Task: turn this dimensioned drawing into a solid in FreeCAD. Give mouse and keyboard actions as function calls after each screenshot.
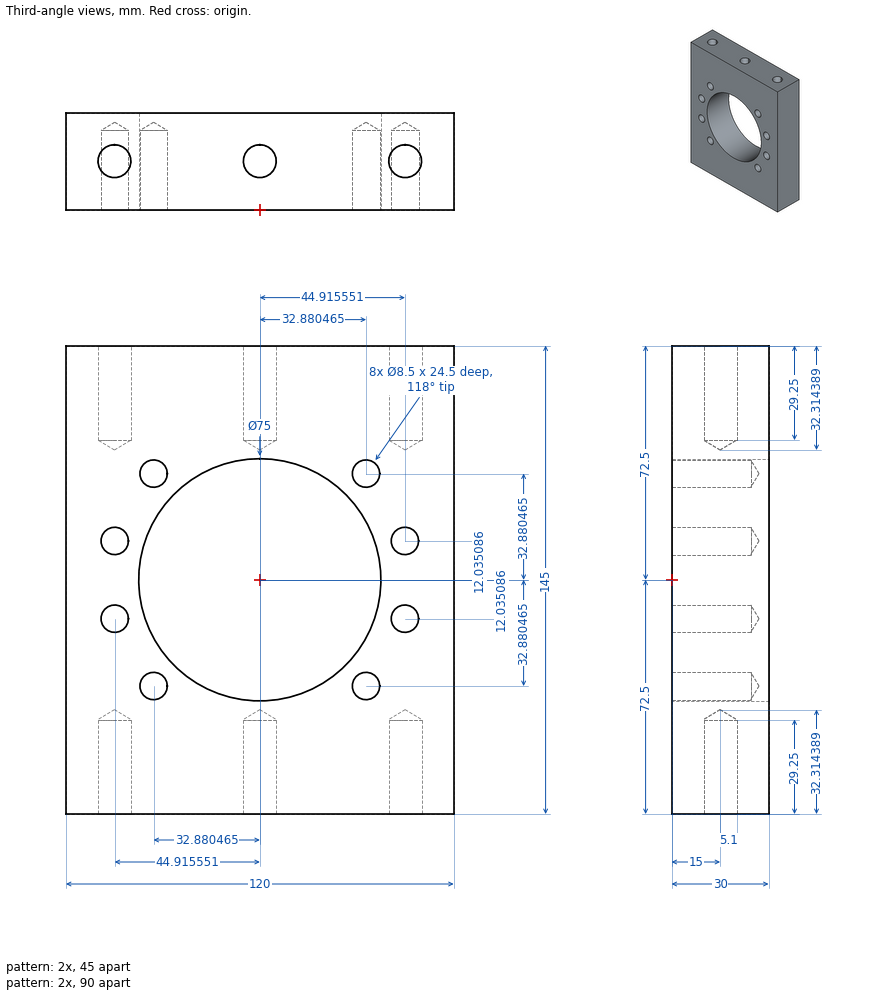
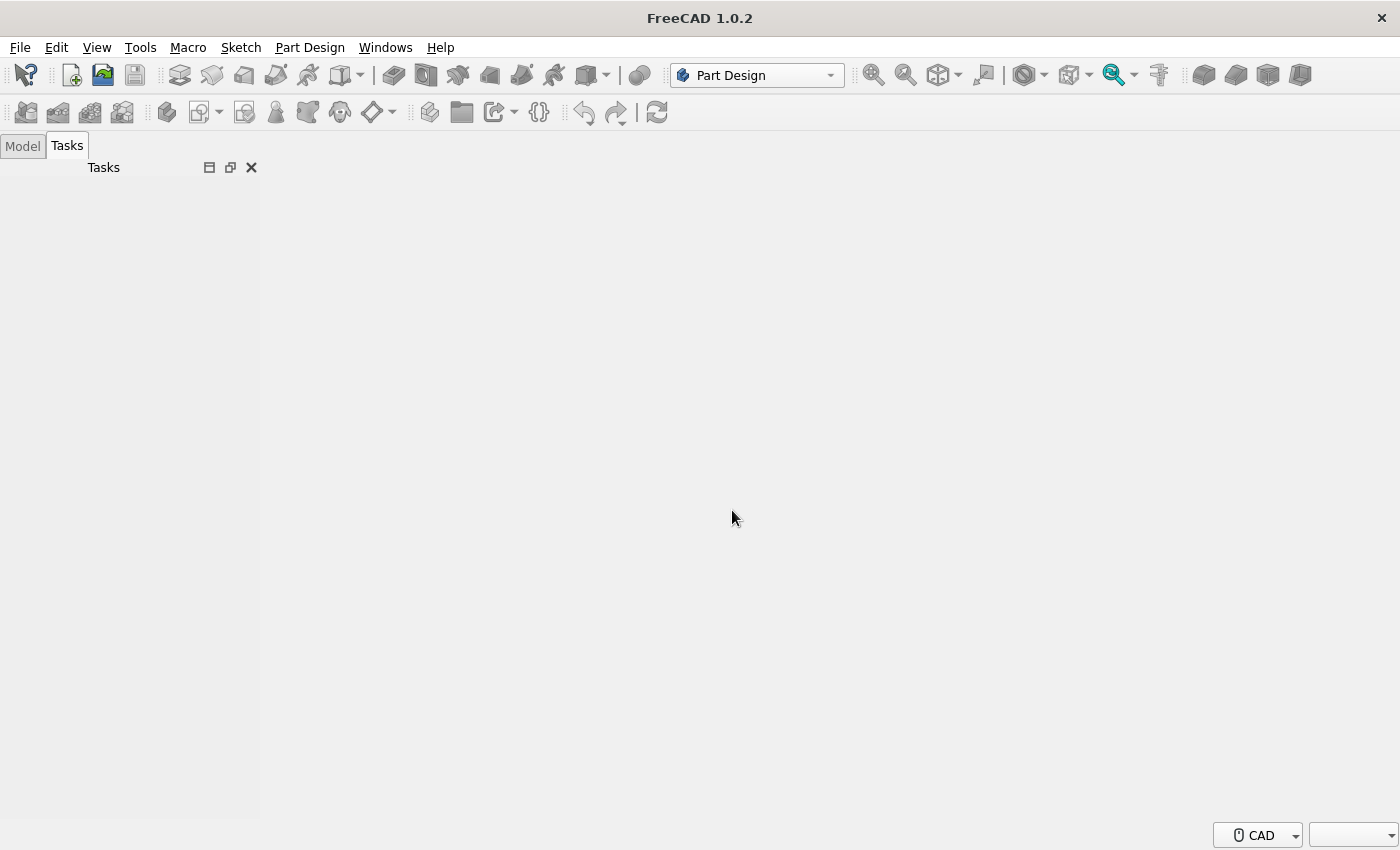
click(72, 76)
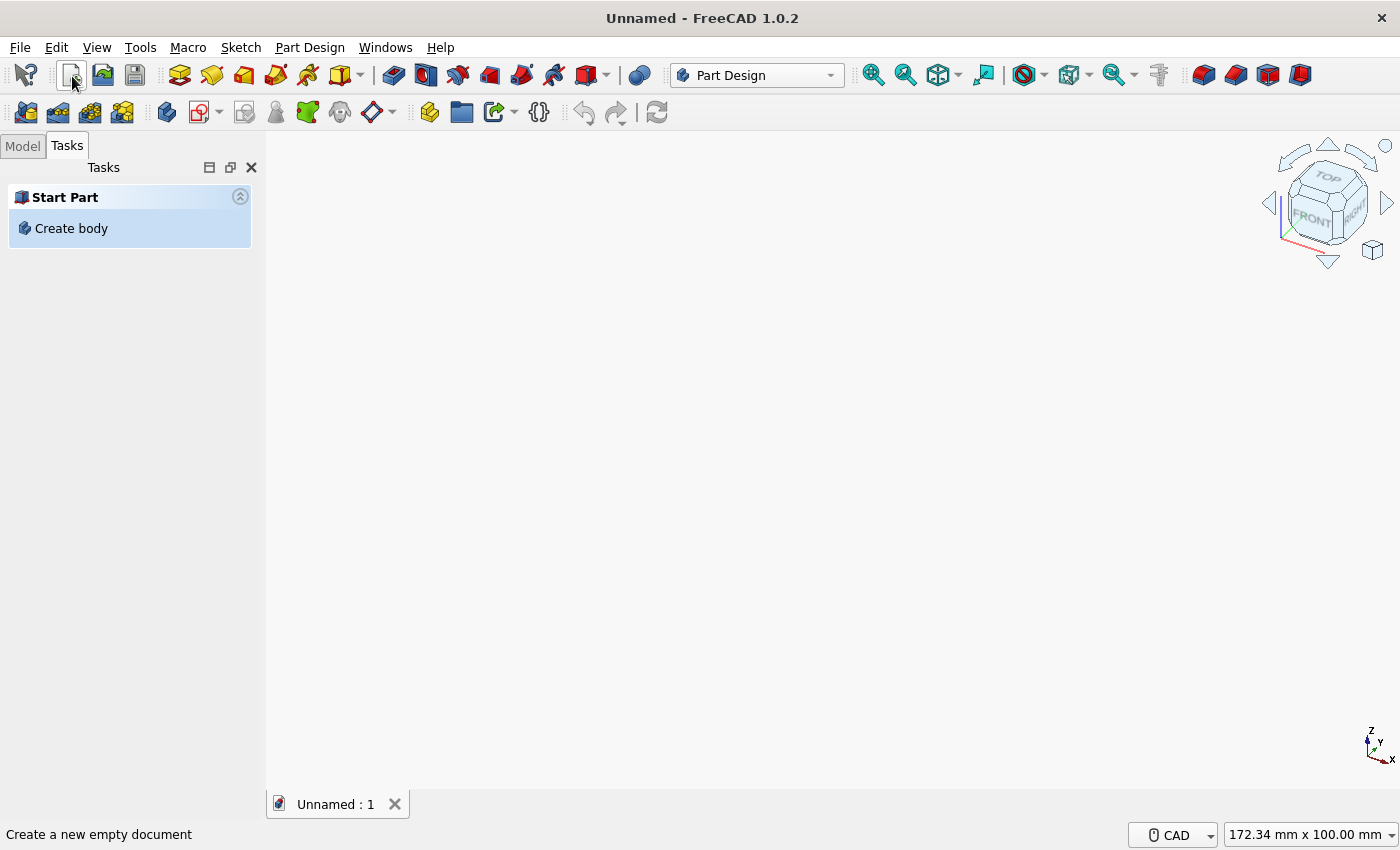
click(200, 112)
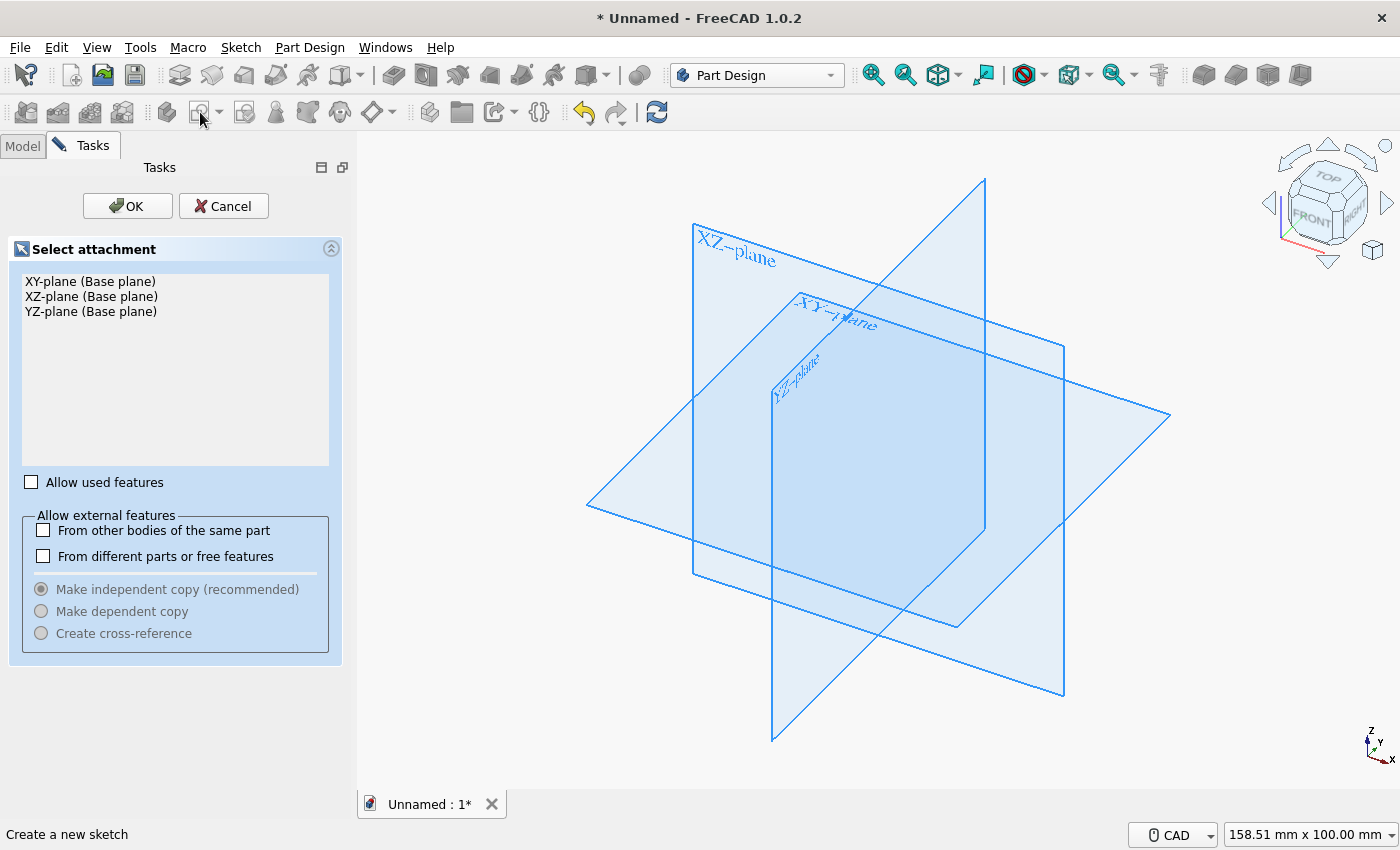
click(82, 296)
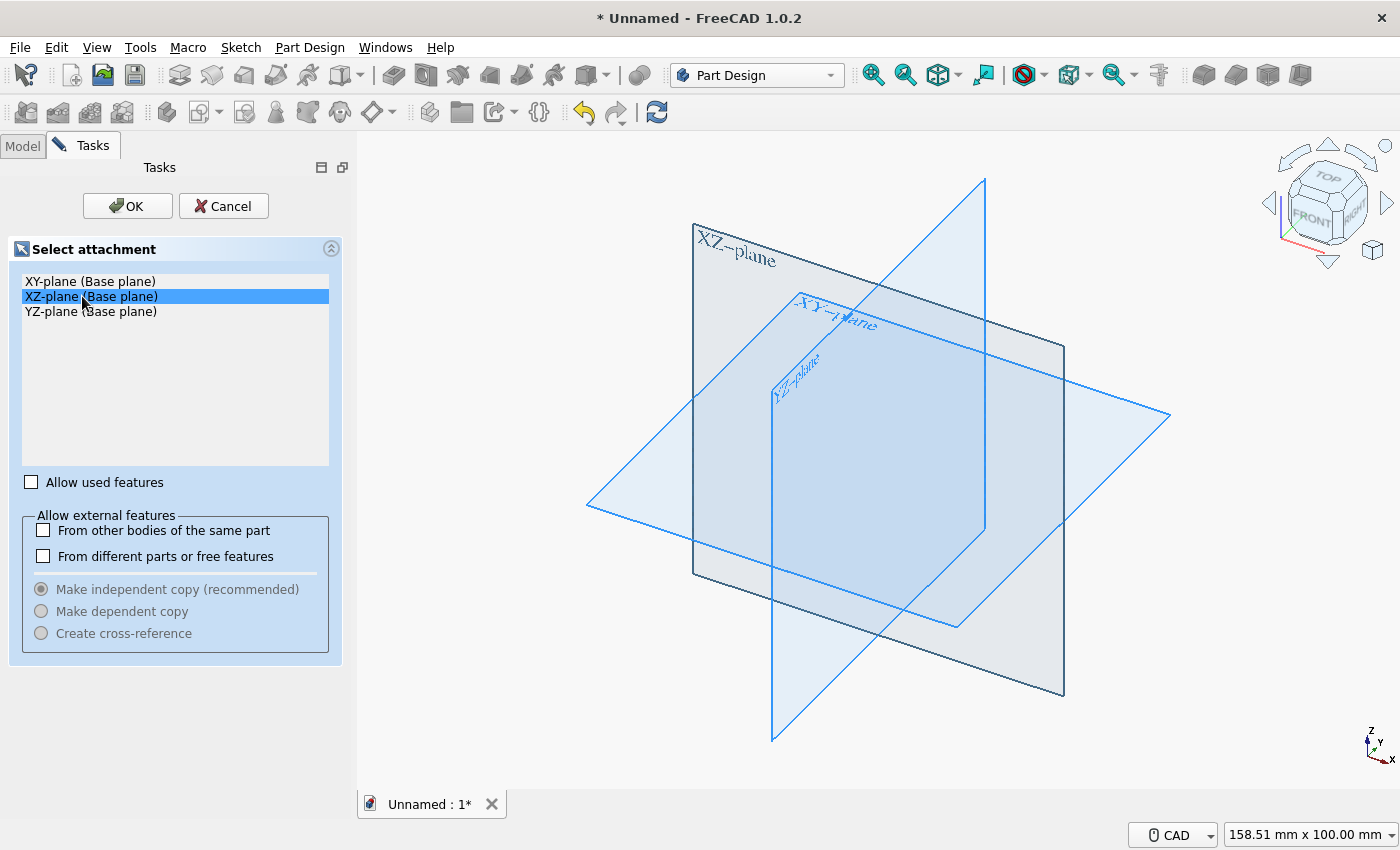
click(128, 206)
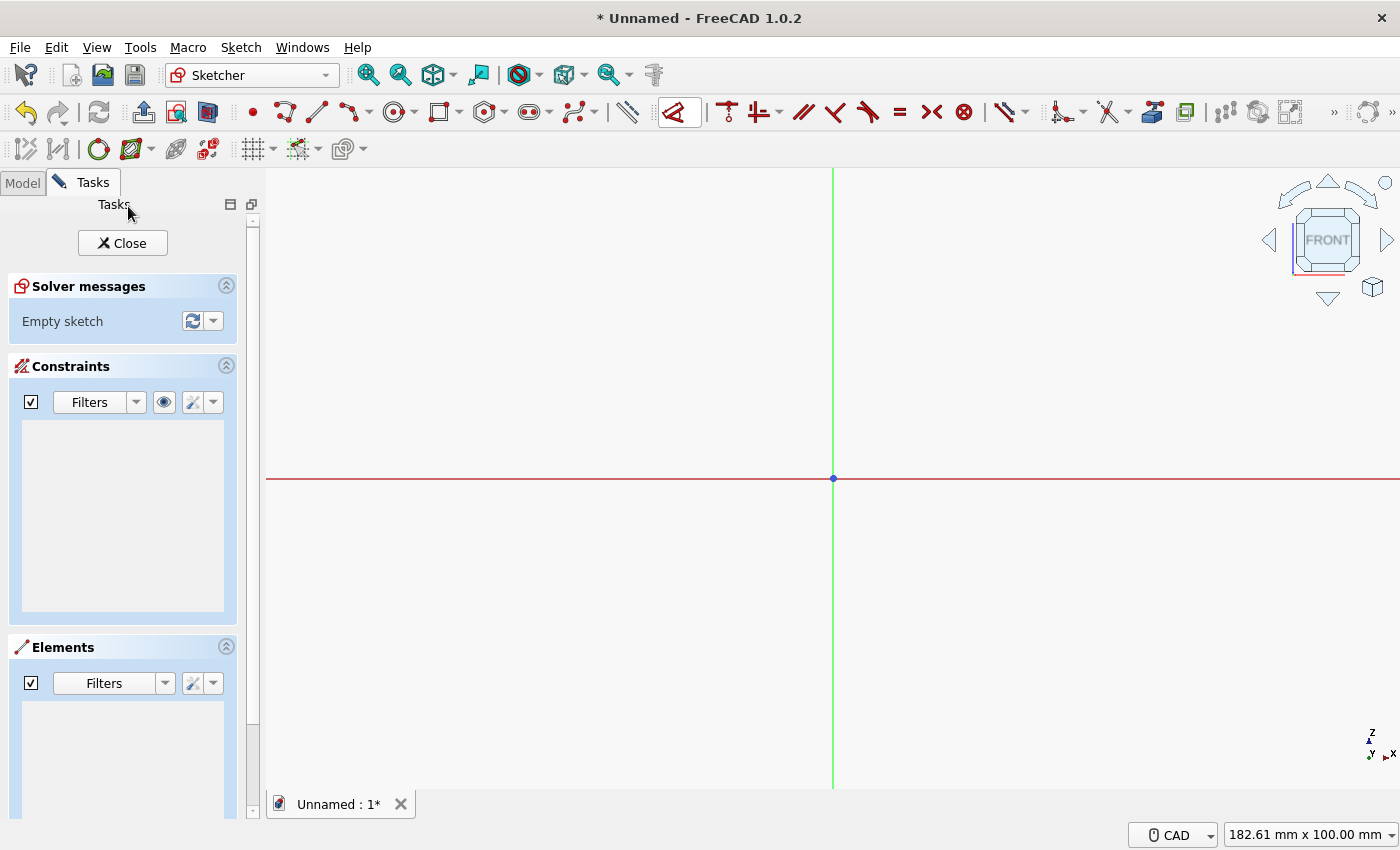
scroll(709, 478, down, 4)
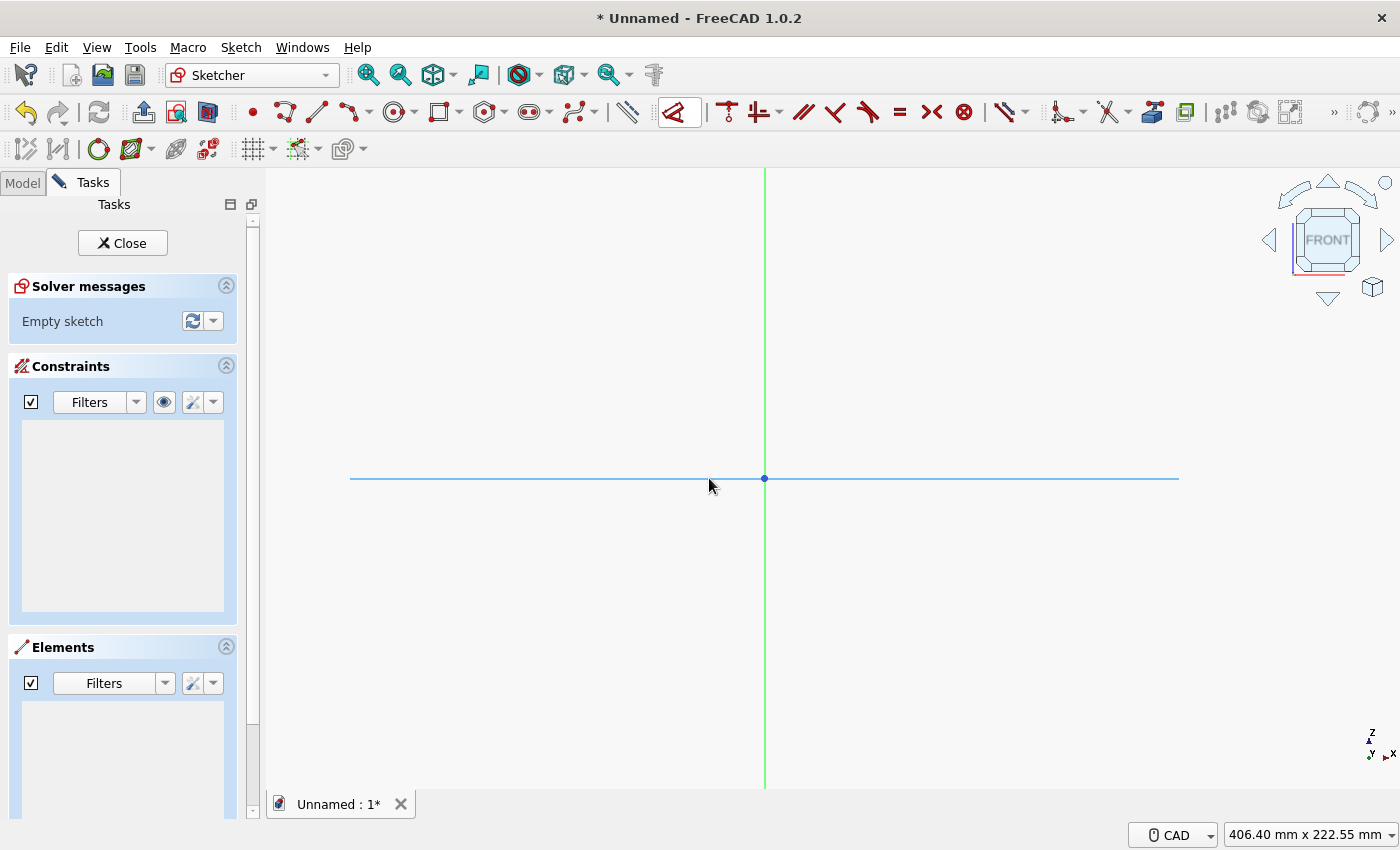
click(462, 112)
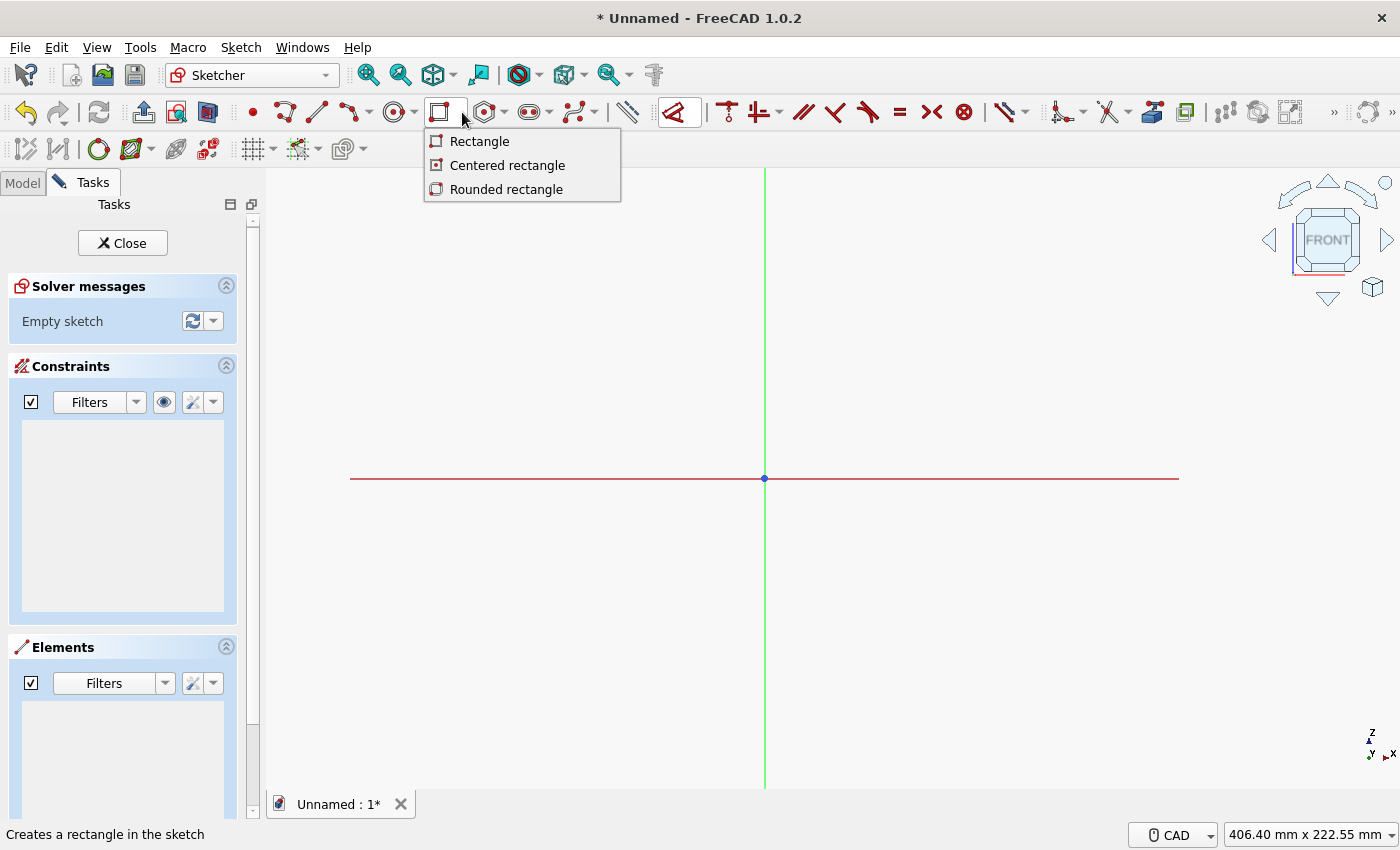
click(522, 165)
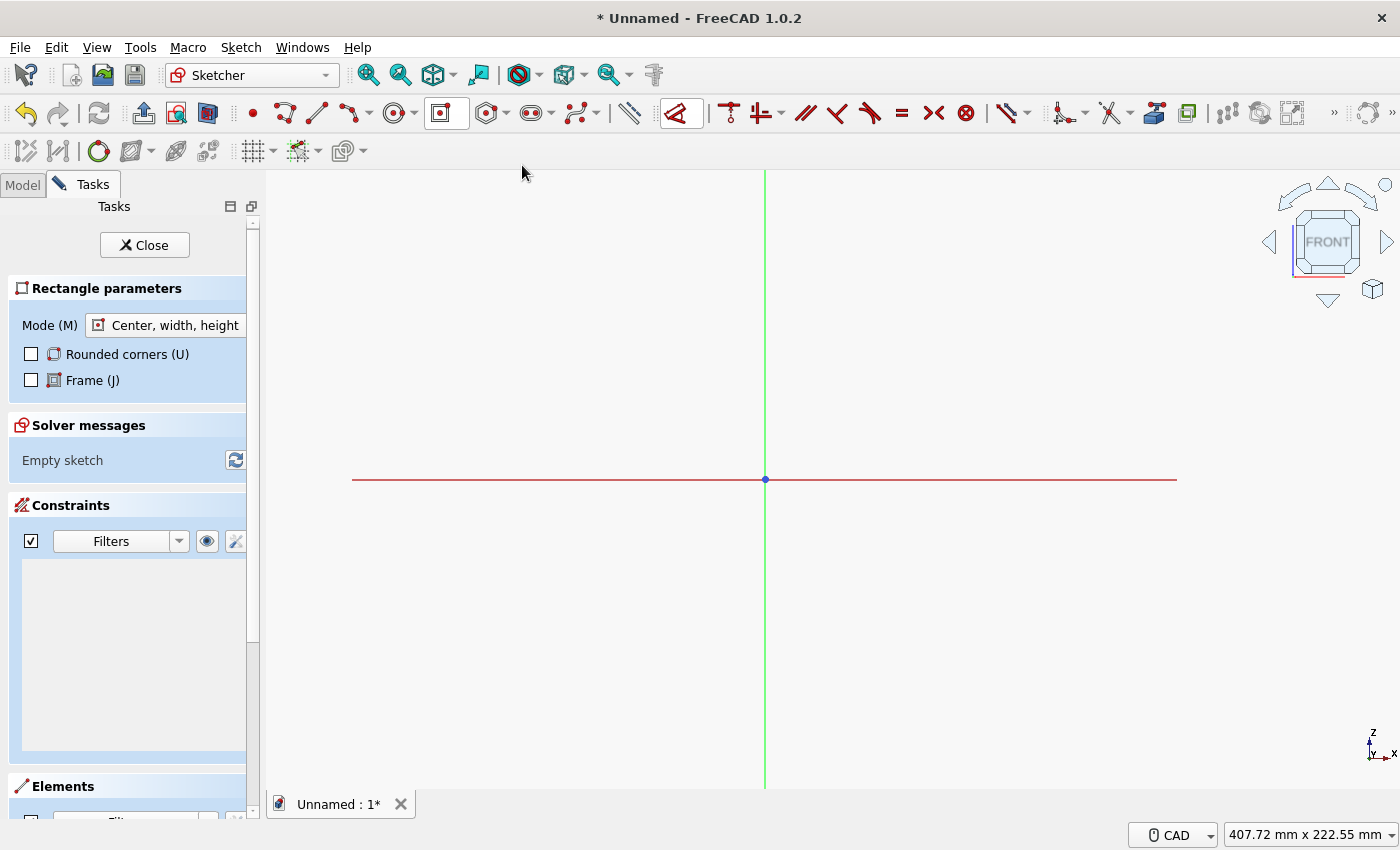
click(765, 480)
click(932, 278)